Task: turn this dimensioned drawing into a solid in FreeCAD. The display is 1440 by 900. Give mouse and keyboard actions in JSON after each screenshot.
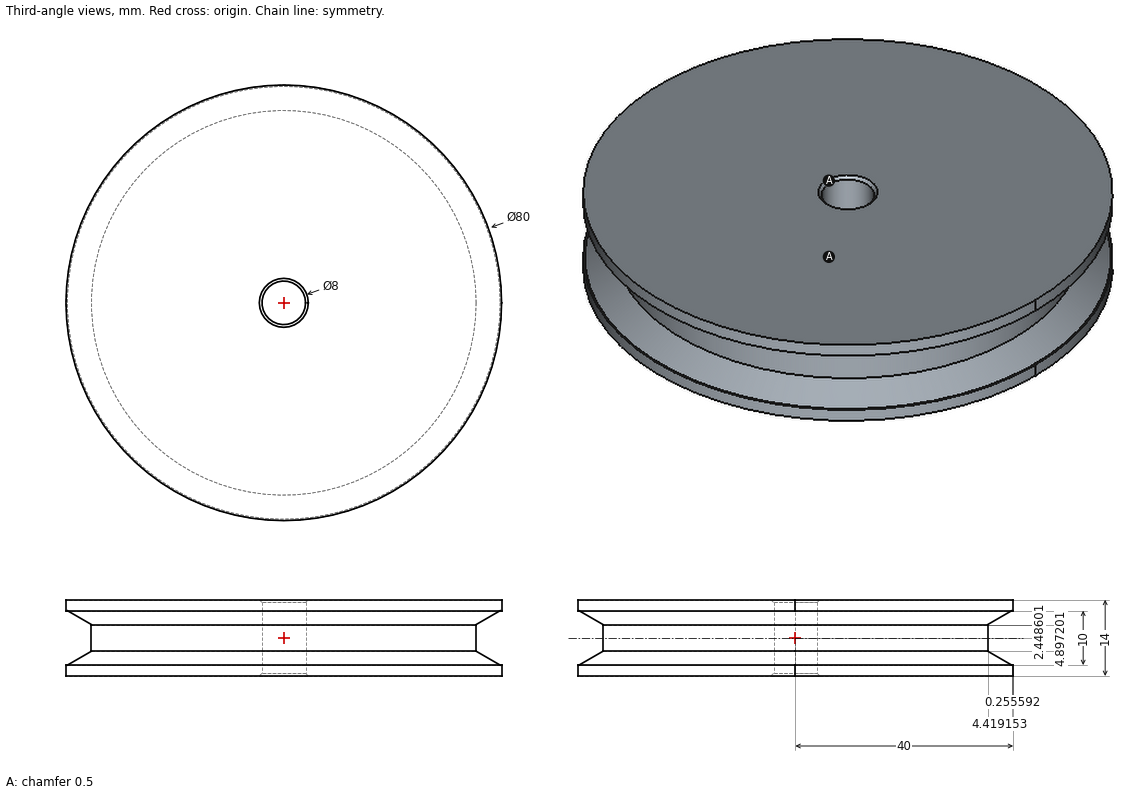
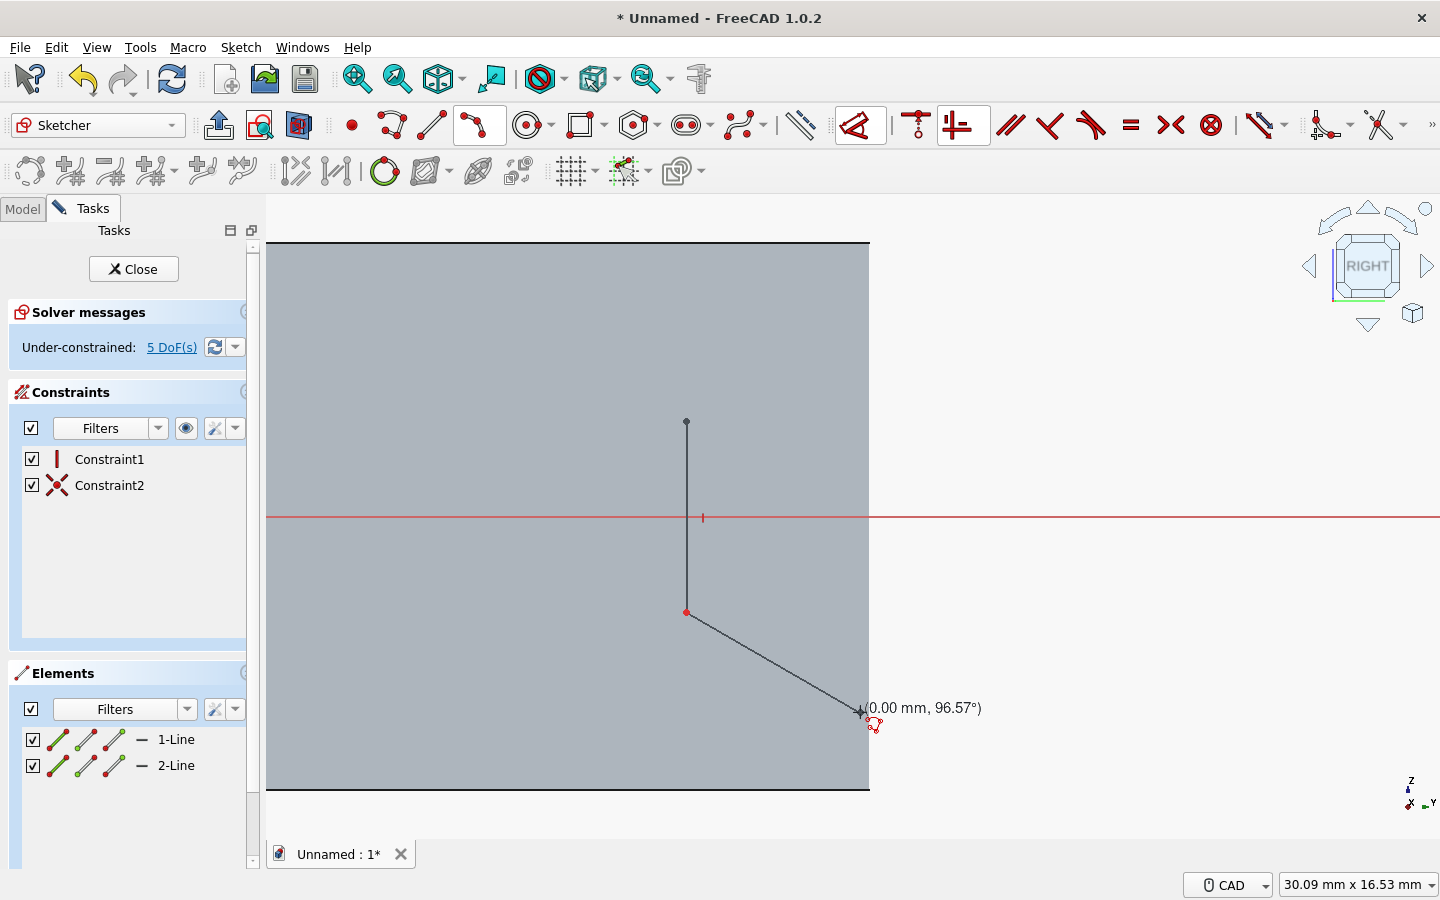
{"action": "scroll", "coordinate": [870, 712], "scroll_direction": "up", "scroll_amount": 3}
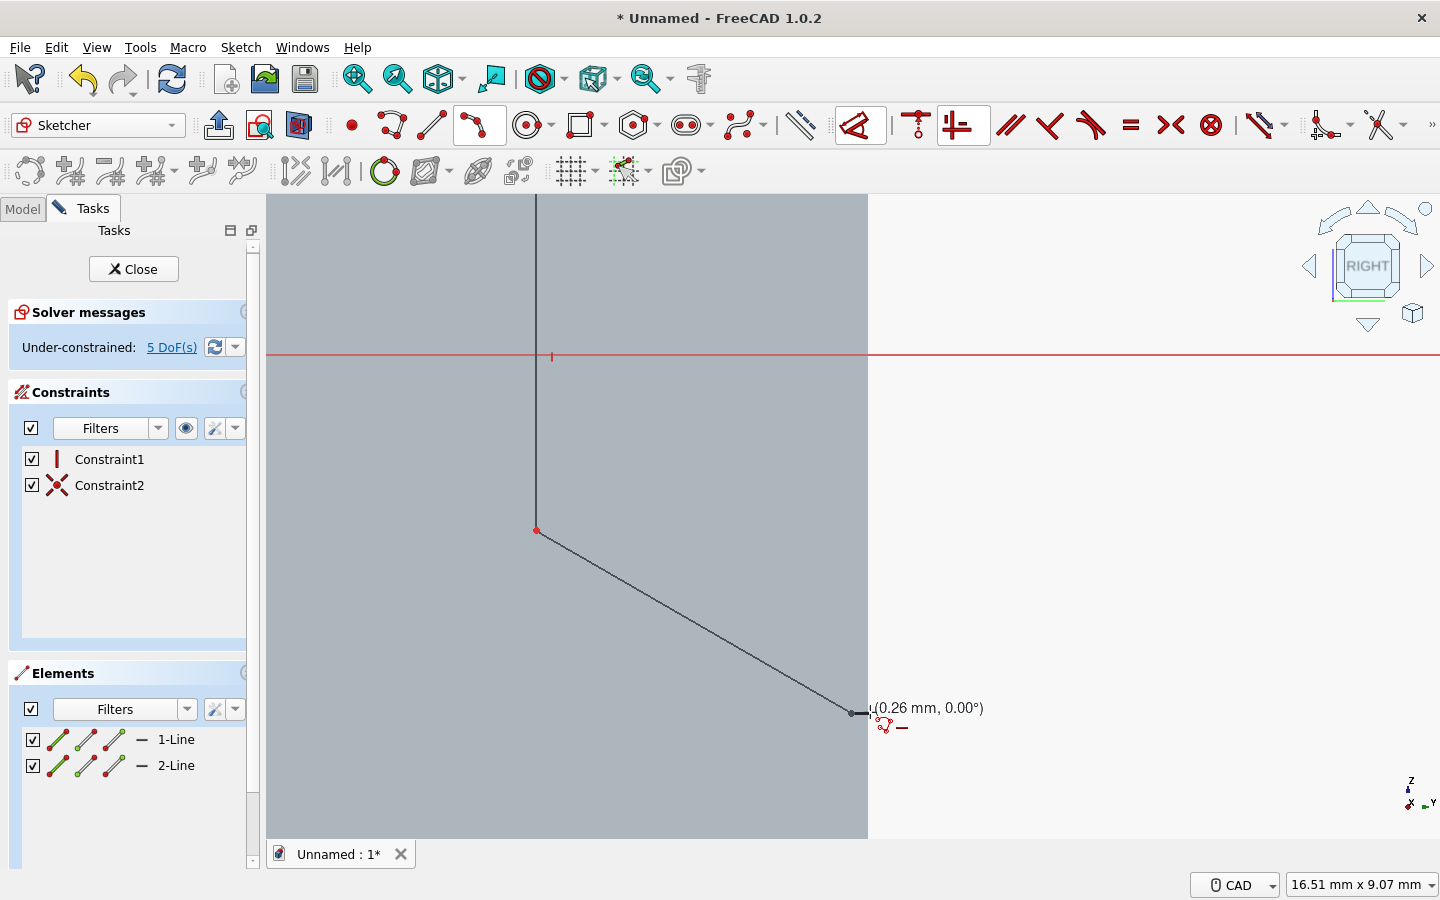
{"action": "left_click", "coordinate": [869, 711]}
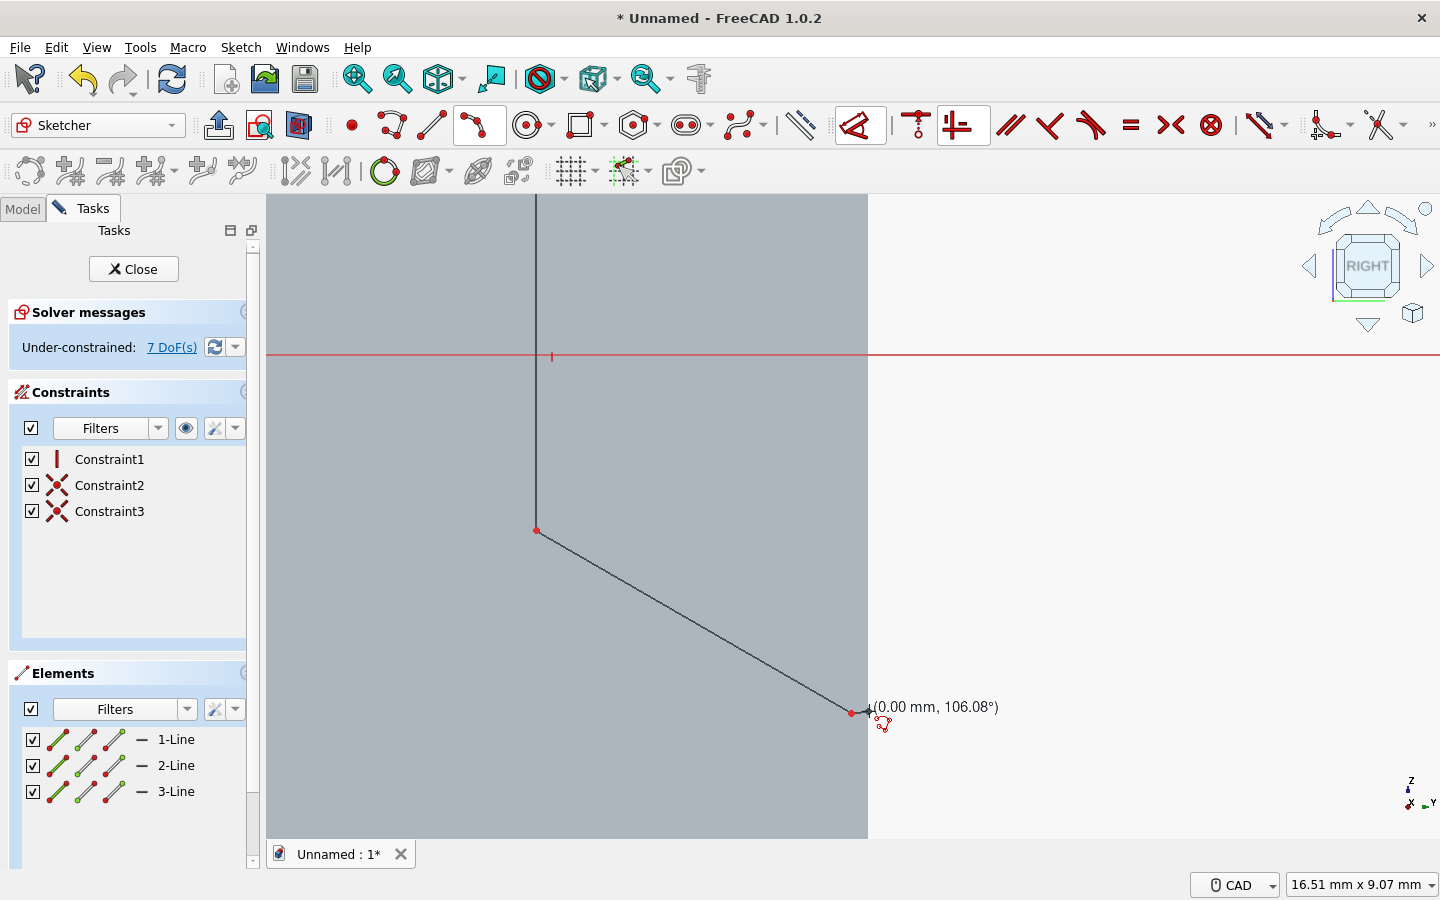
{"action": "scroll", "coordinate": [884, 713], "scroll_direction": "down", "scroll_amount": 3}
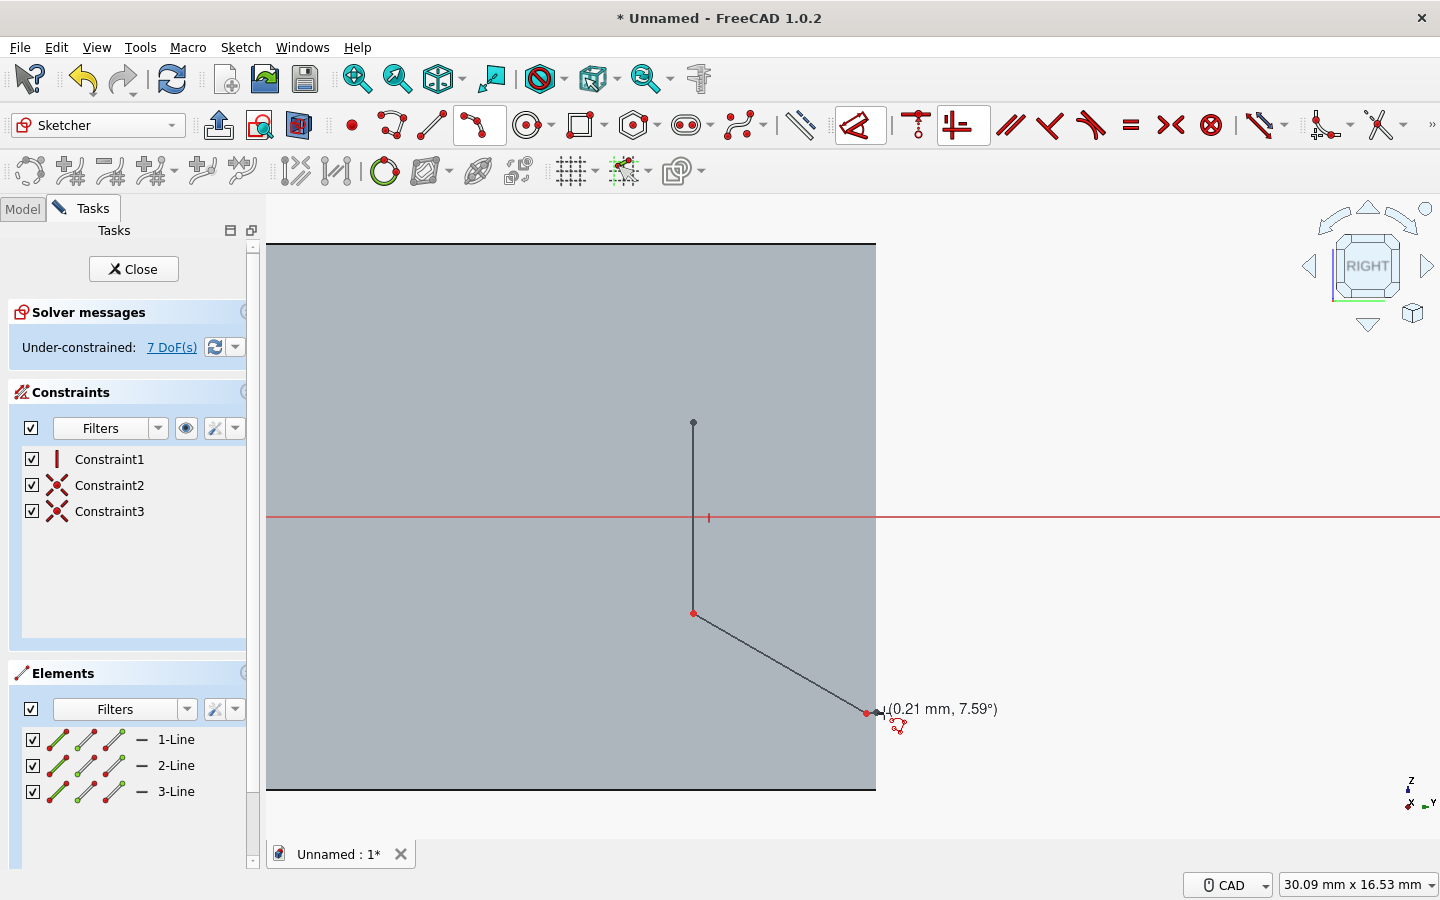
{"action": "left_click", "coordinate": [876, 322]}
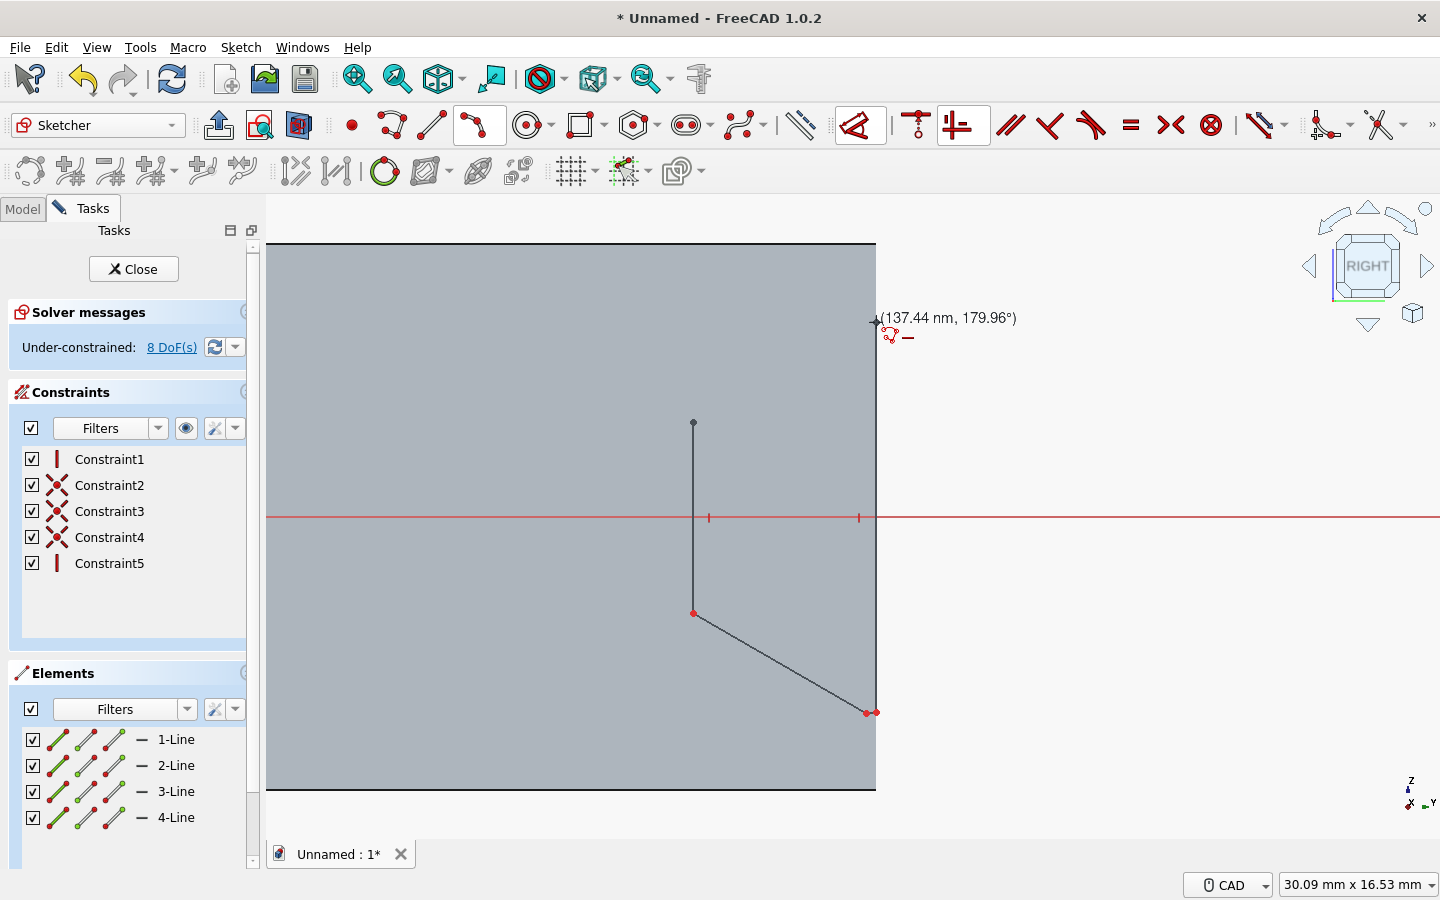
{"action": "scroll", "coordinate": [866, 322], "scroll_direction": "up", "scroll_amount": 3}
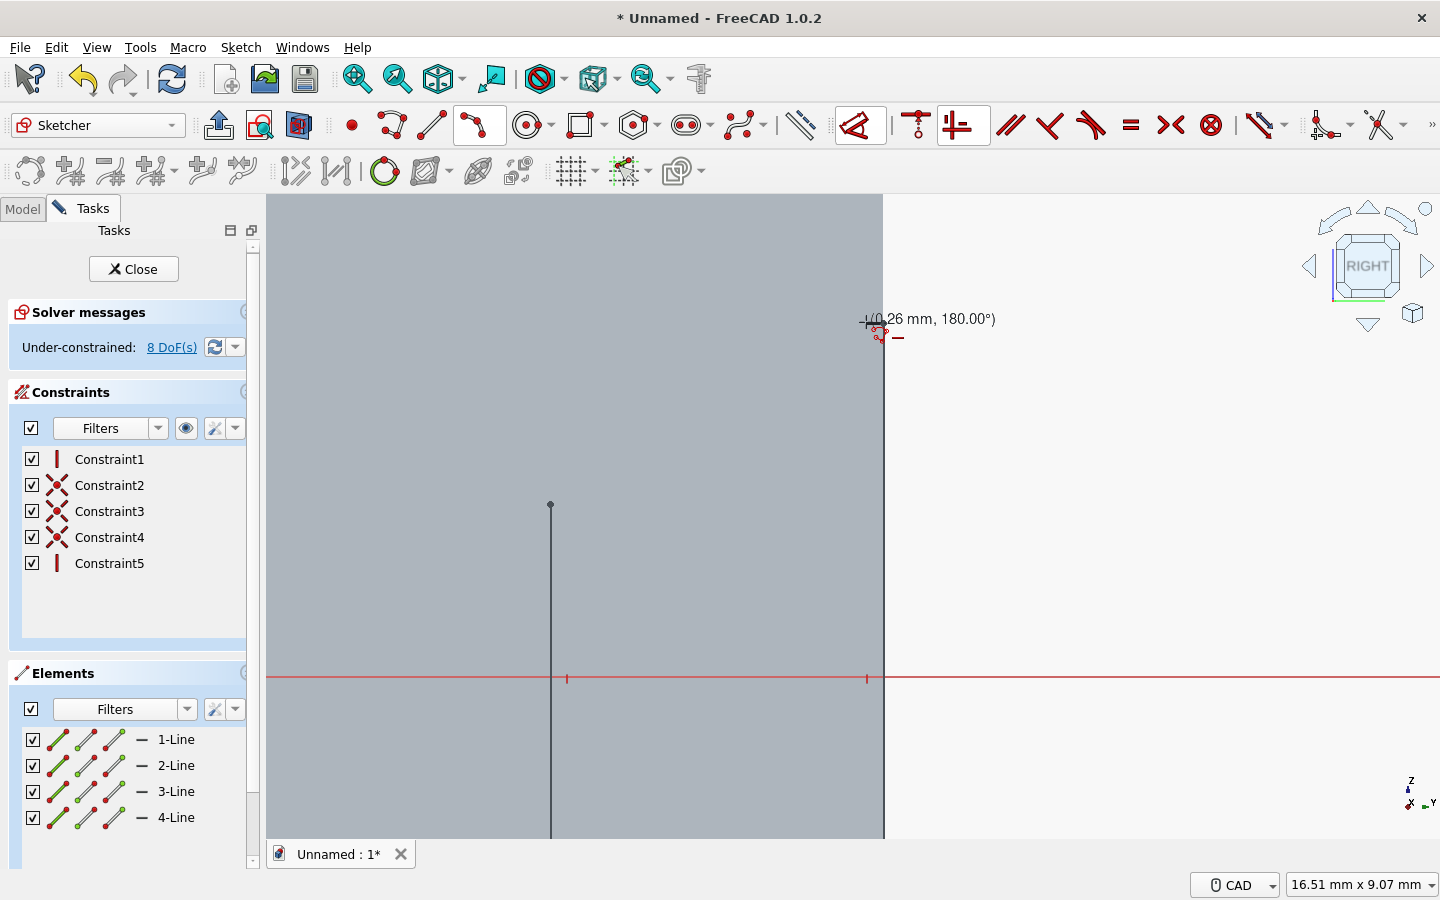
{"action": "left_click", "coordinate": [866, 322]}
{"action": "left_click", "coordinate": [551, 505]}
{"action": "key", "text": "Escape"}
{"action": "key", "text": "Escape"}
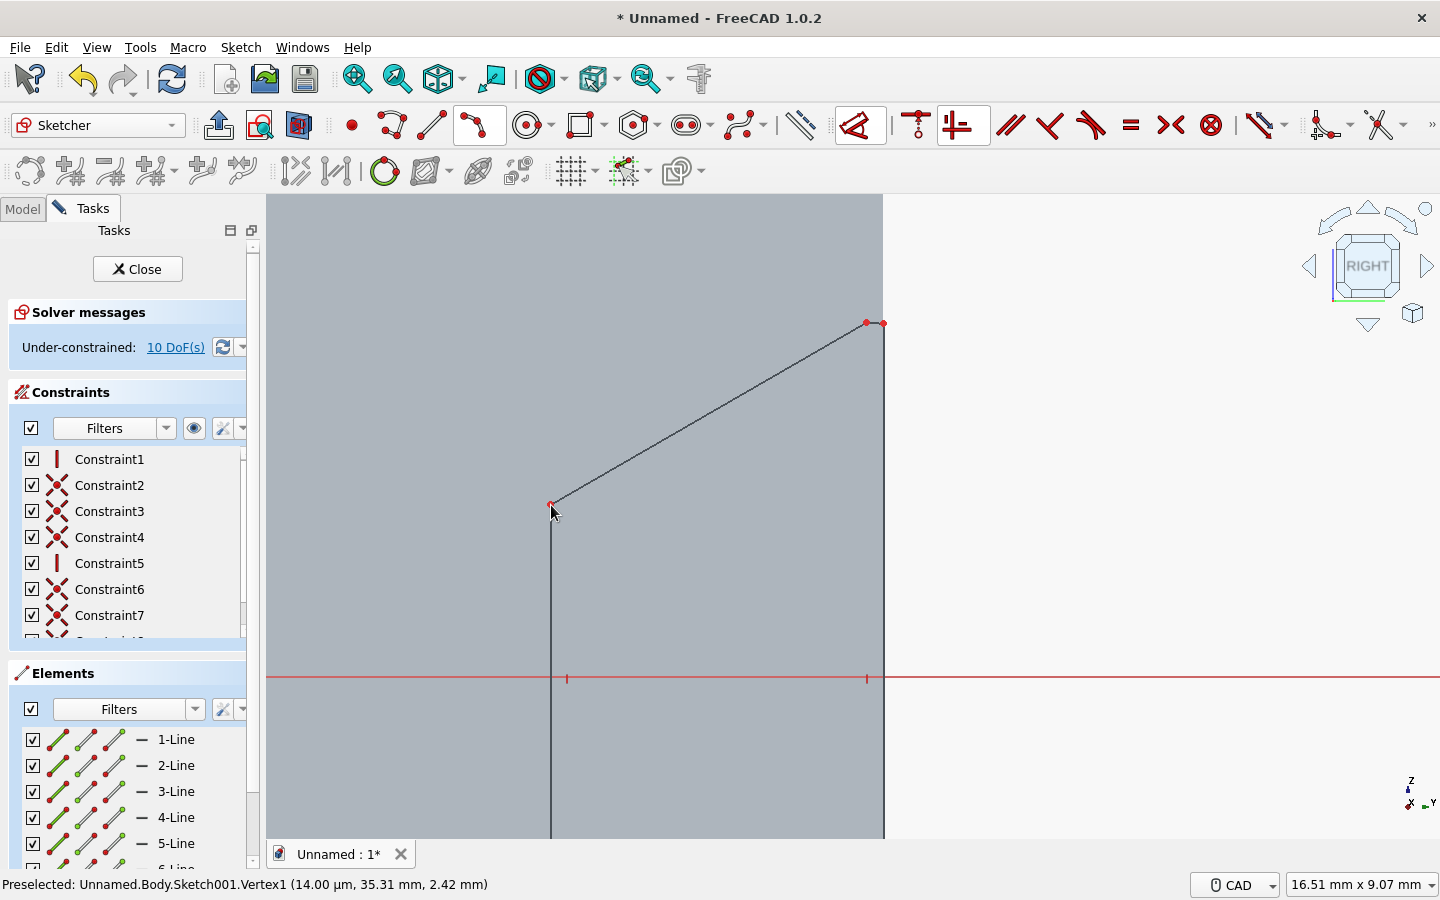
{"action": "scroll", "coordinate": [866, 321], "scroll_direction": "down", "scroll_amount": 3}